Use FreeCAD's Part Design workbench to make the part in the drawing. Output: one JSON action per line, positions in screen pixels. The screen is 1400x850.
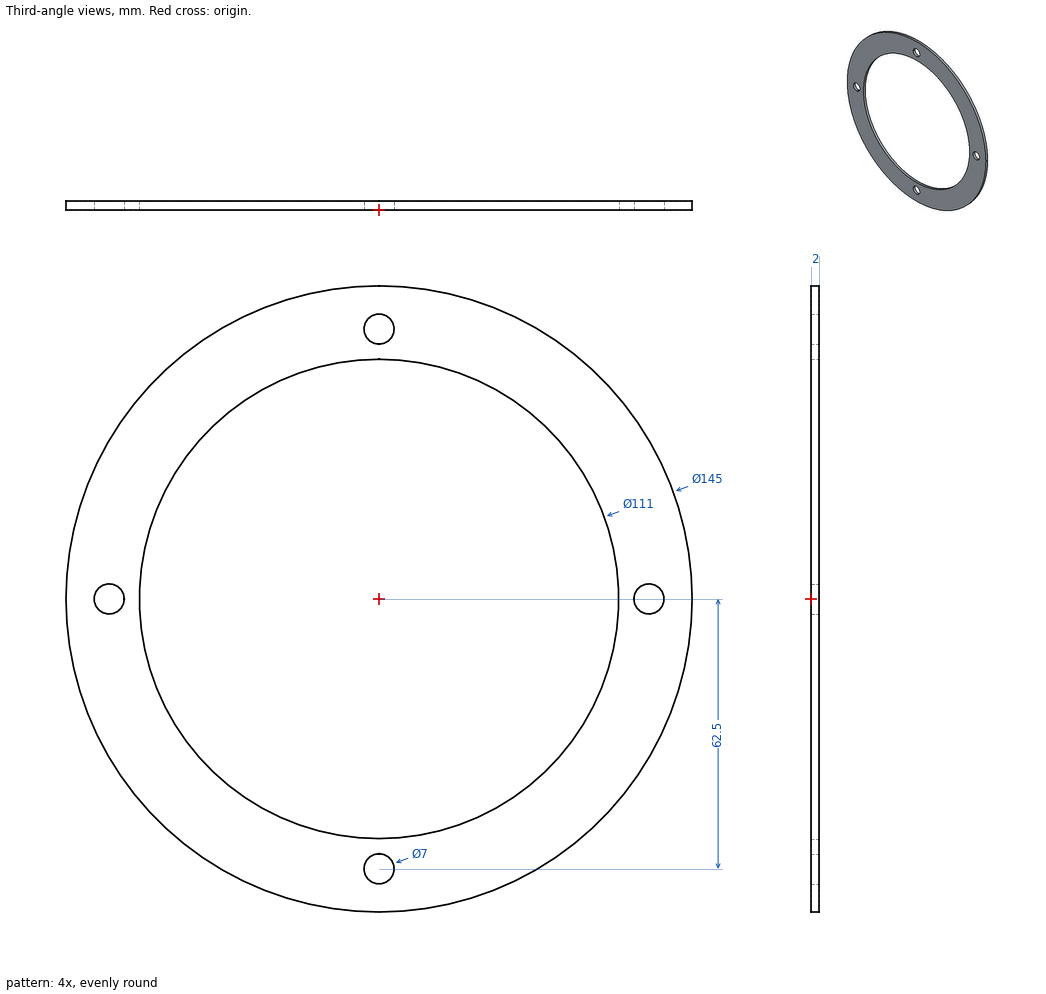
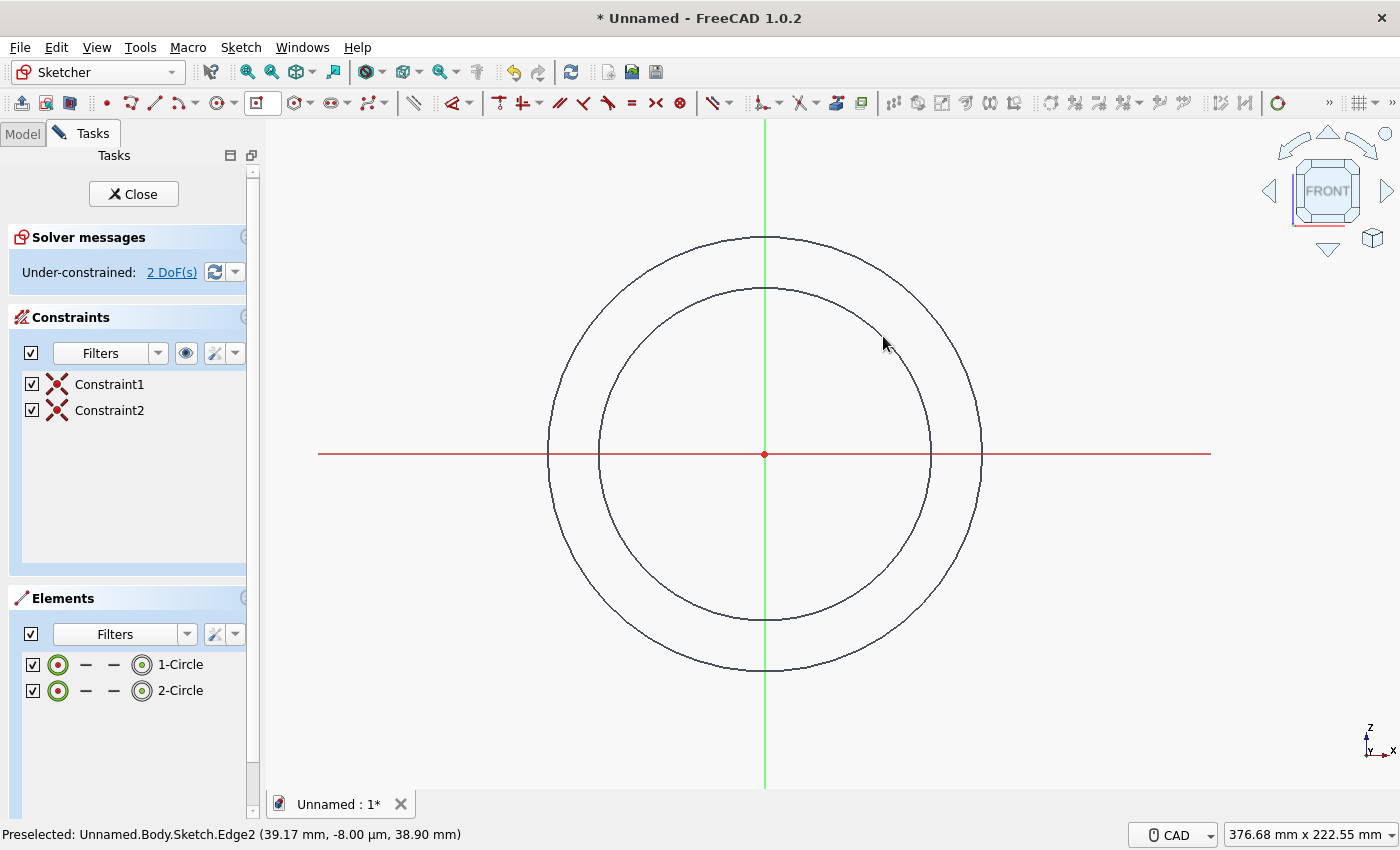
{"action": "left_click", "coordinate": [452, 104]}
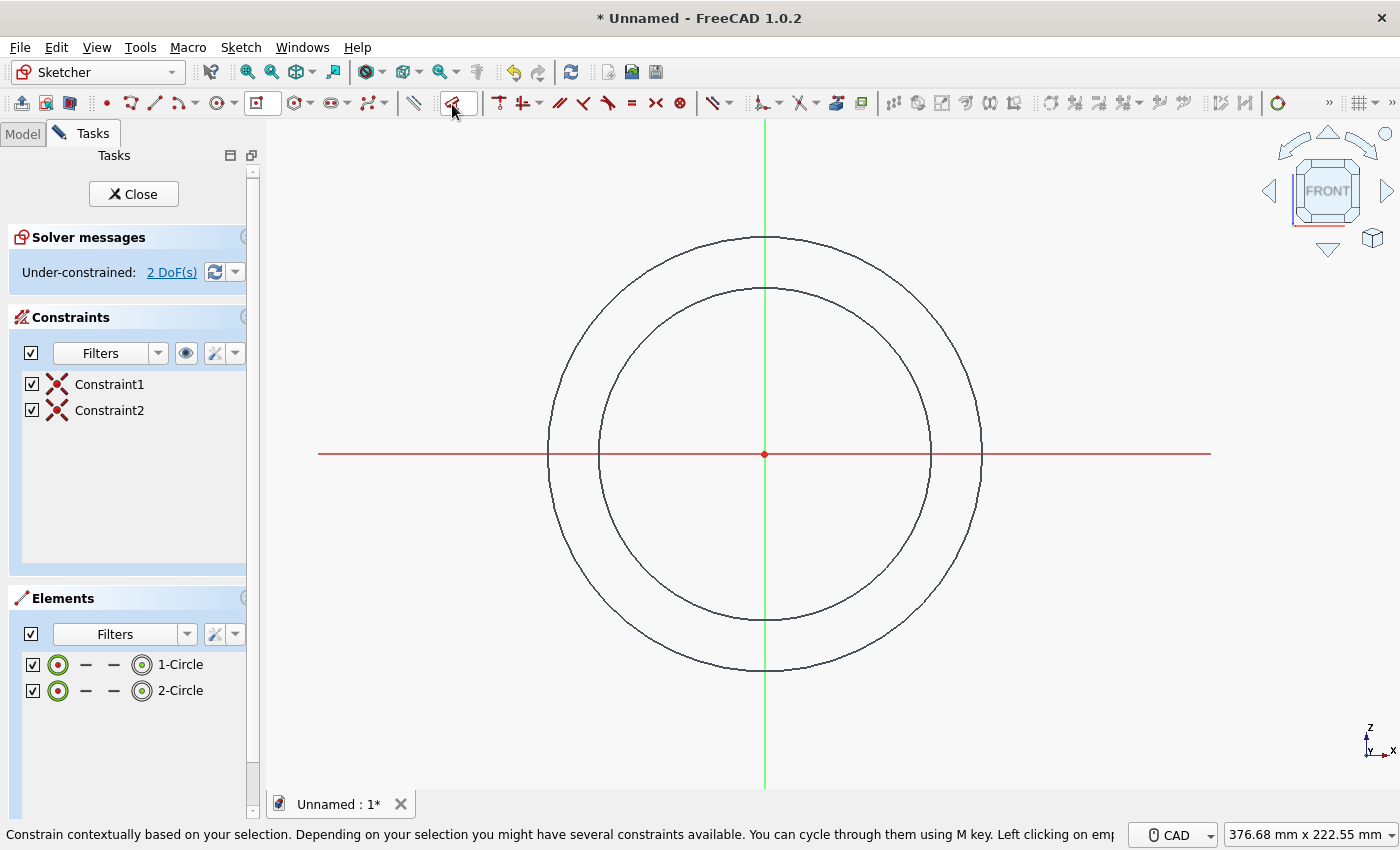
{"action": "left_click", "coordinate": [918, 300]}
{"action": "left_click", "coordinate": [941, 277]}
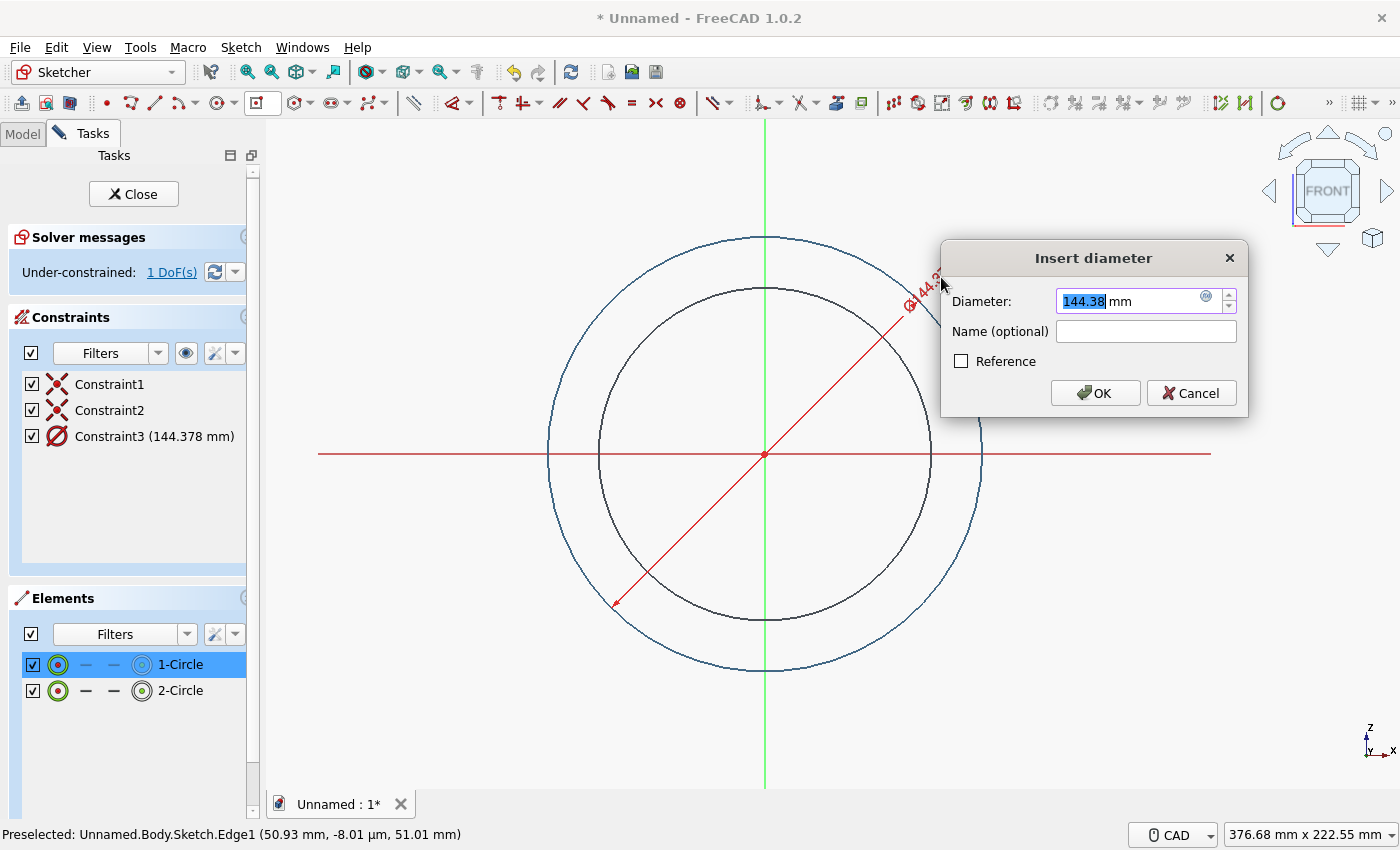
{"action": "type", "text": "145"}
{"action": "key", "text": "Return"}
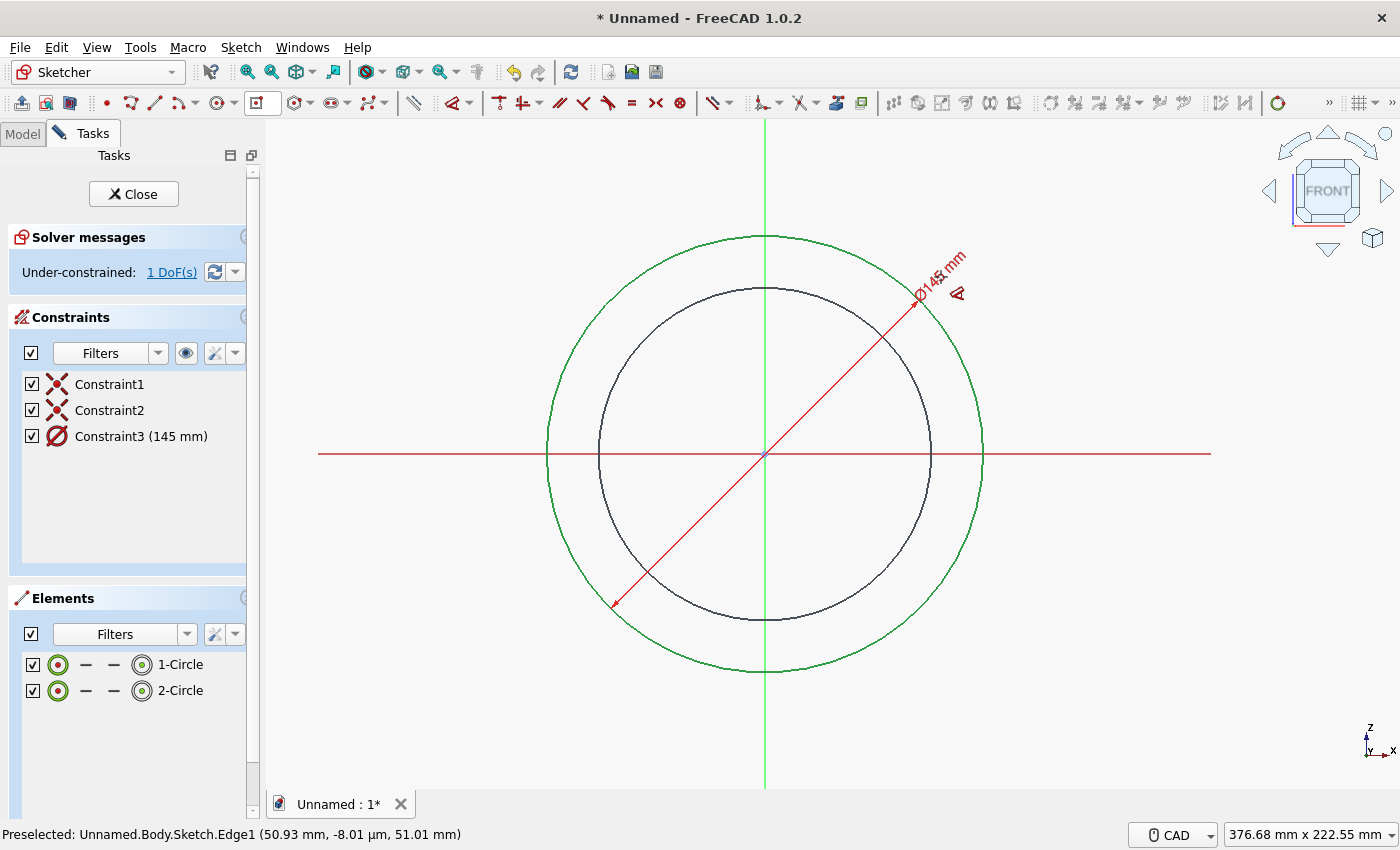
{"action": "left_click", "coordinate": [882, 336]}
{"action": "left_click", "coordinate": [905, 313]}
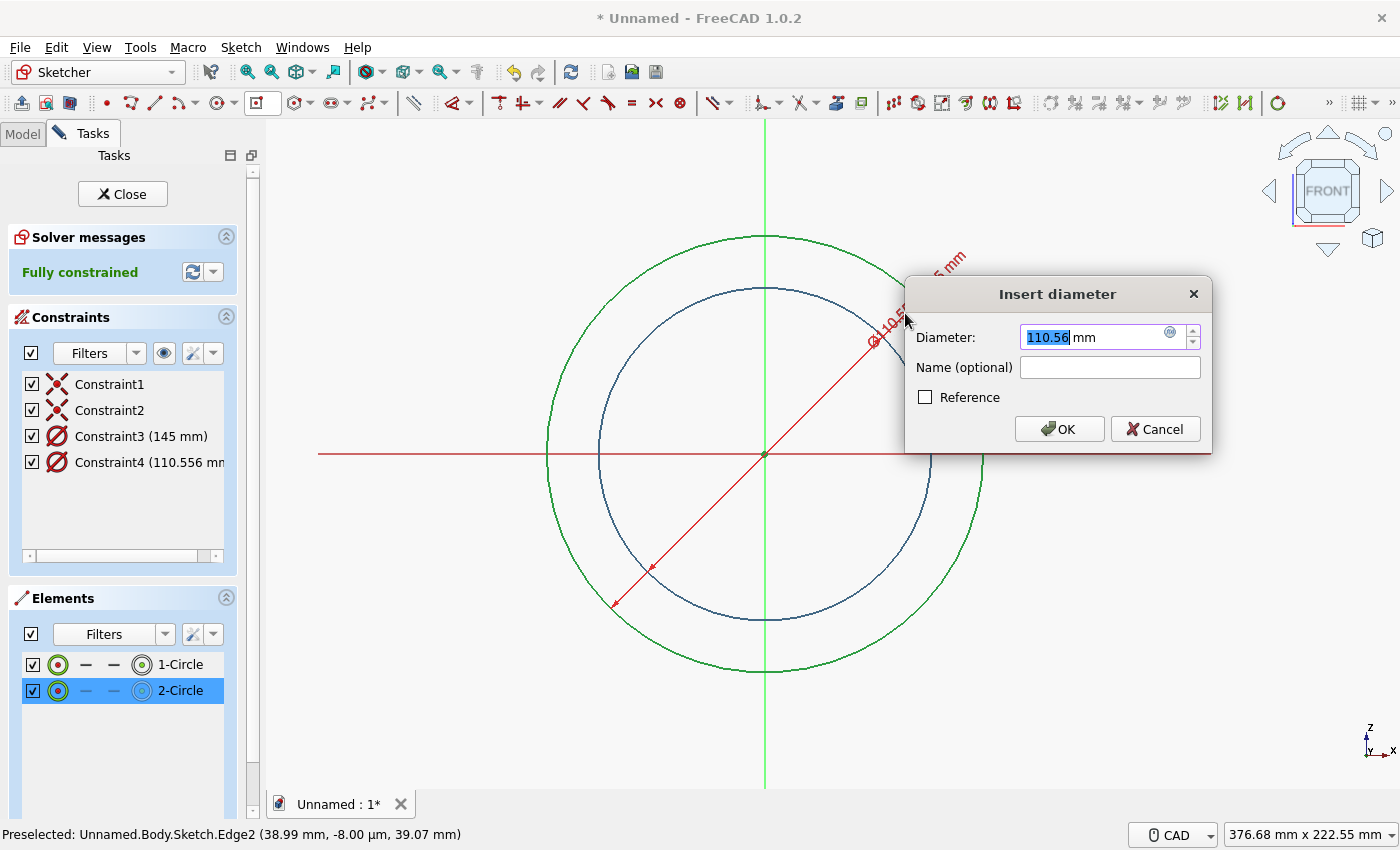
{"action": "type", "text": "111"}
{"action": "key", "text": "Return"}
{"action": "key", "text": "Escape"}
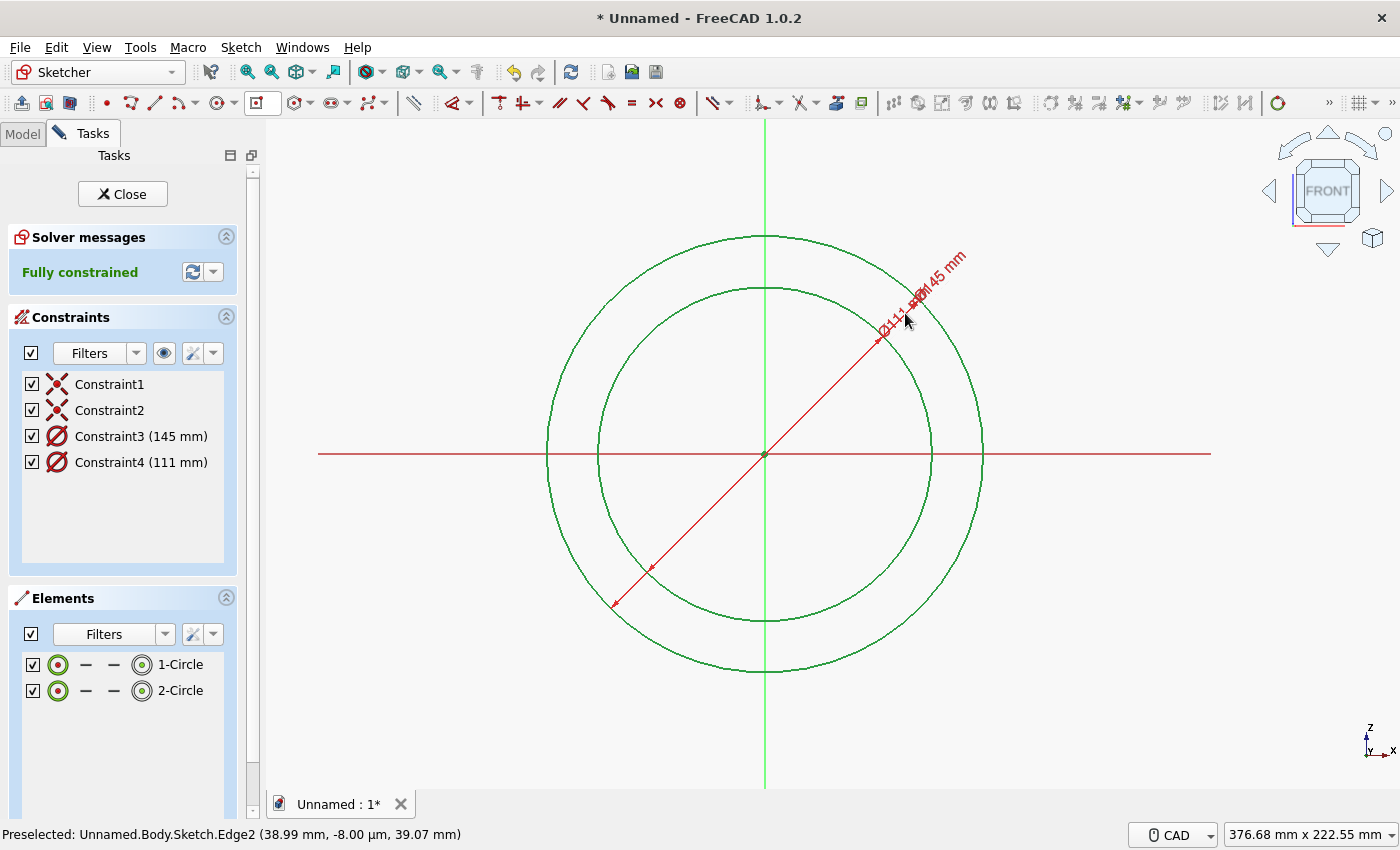
{"action": "left_click", "coordinate": [123, 194]}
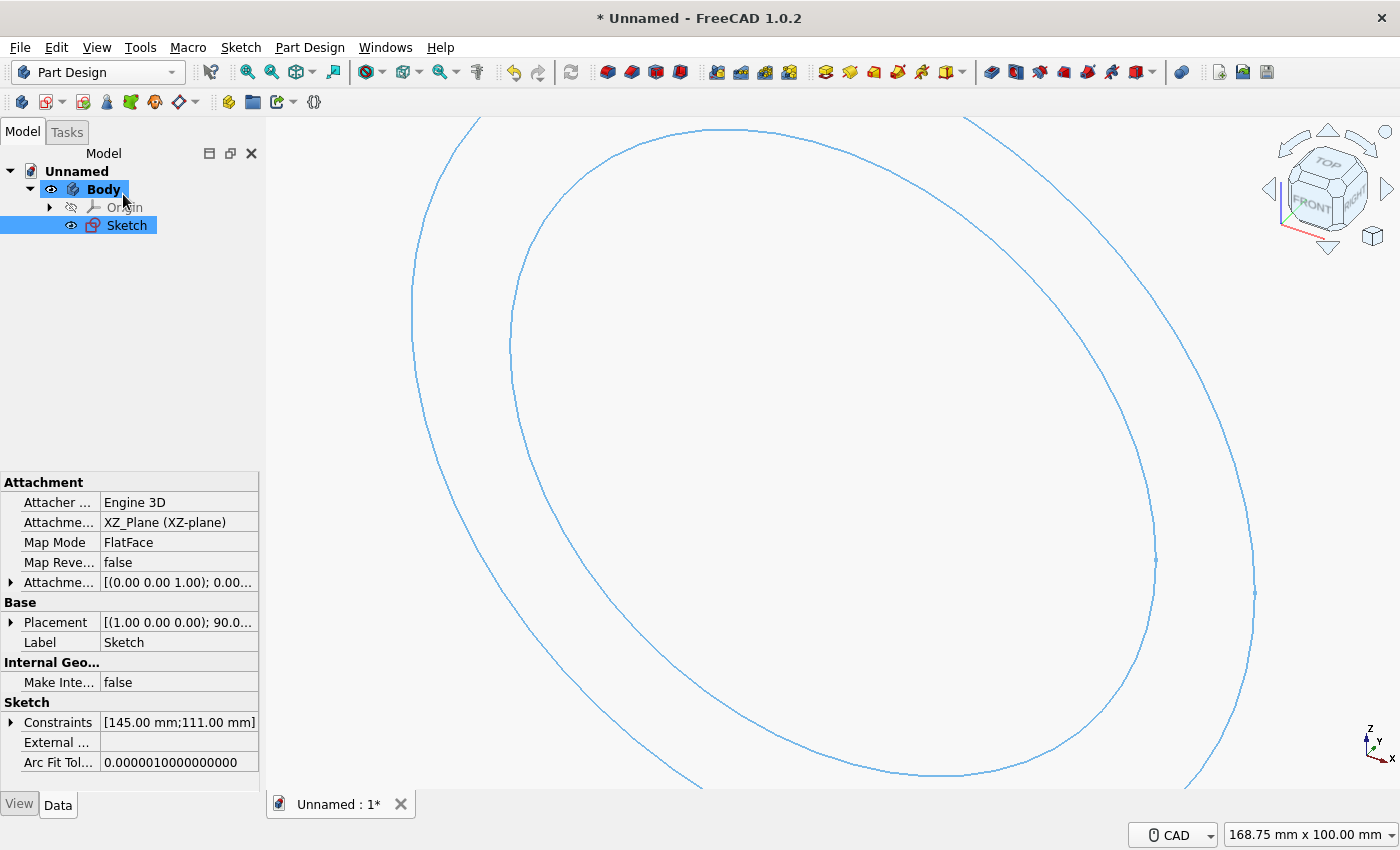
{"action": "left_click", "coordinate": [826, 72]}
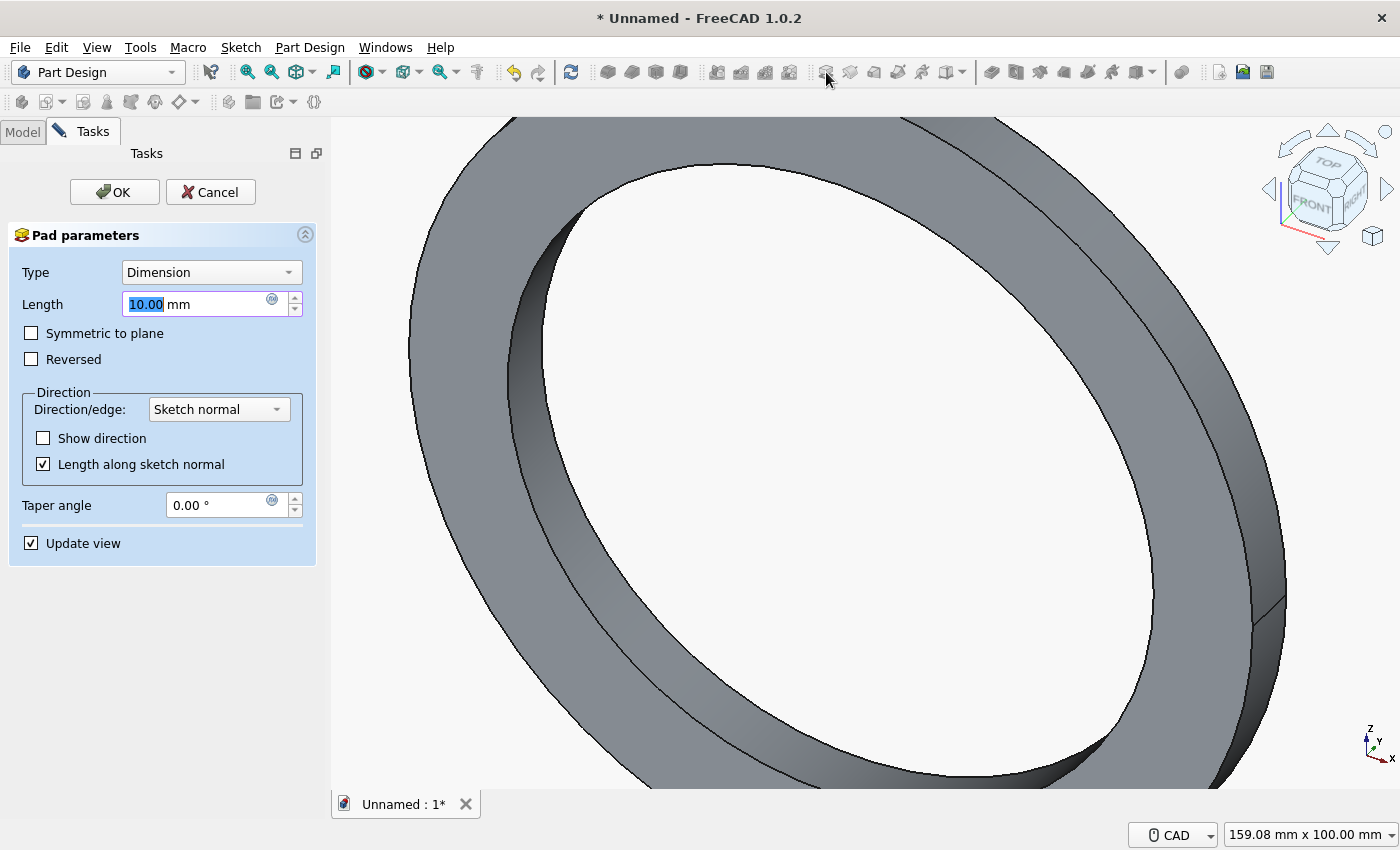
{"action": "type", "text": "2"}
{"action": "key", "text": "Tab"}